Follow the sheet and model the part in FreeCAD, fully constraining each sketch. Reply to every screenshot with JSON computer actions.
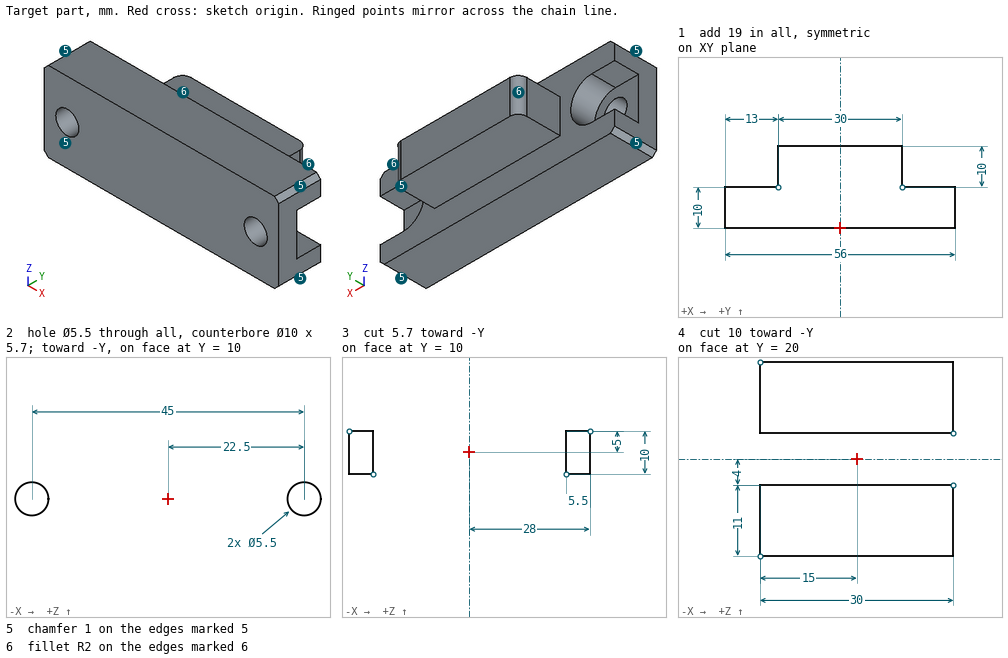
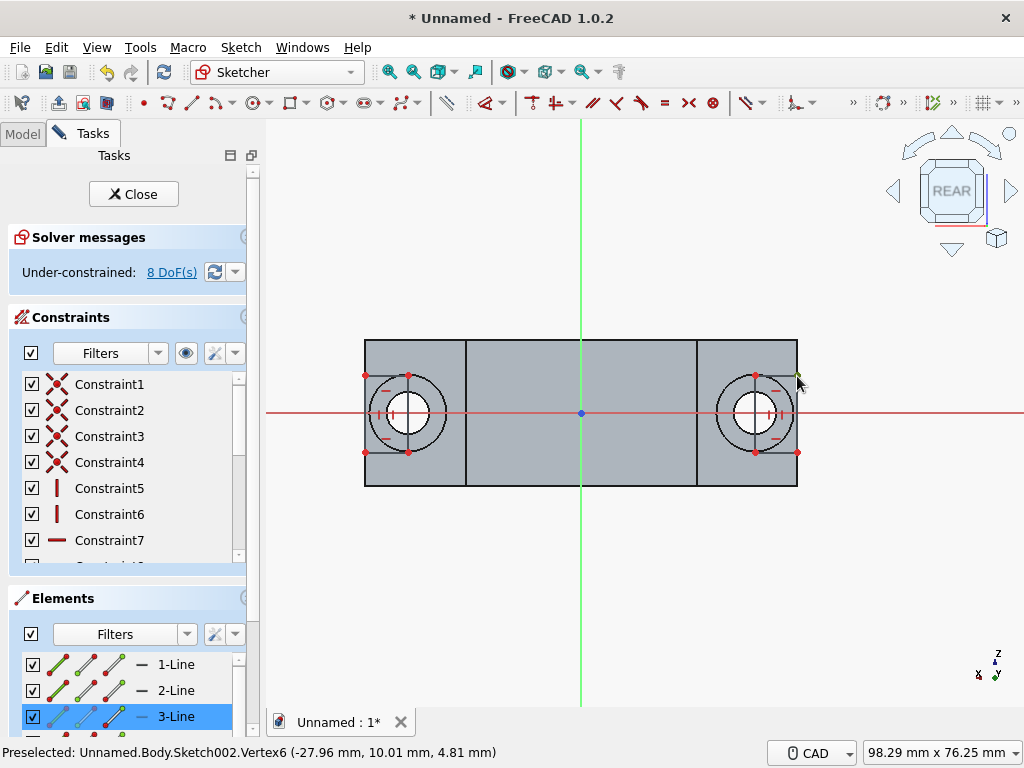
{"action": "left_click", "coordinate": [365, 376]}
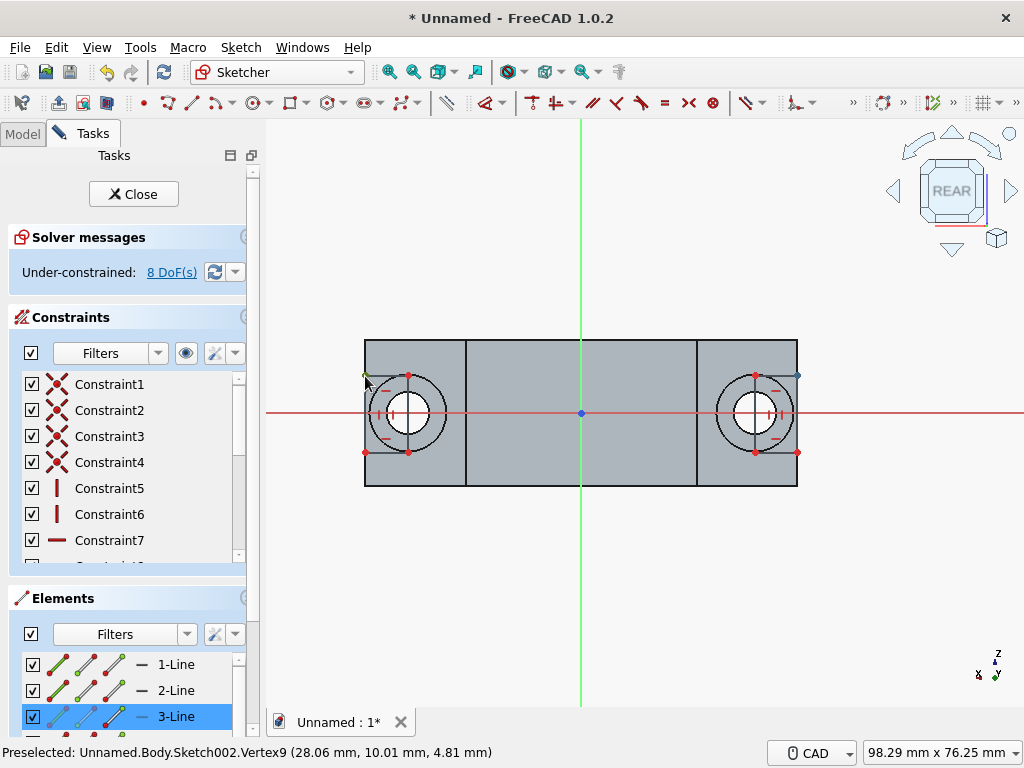
{"action": "left_click", "coordinate": [581, 641]}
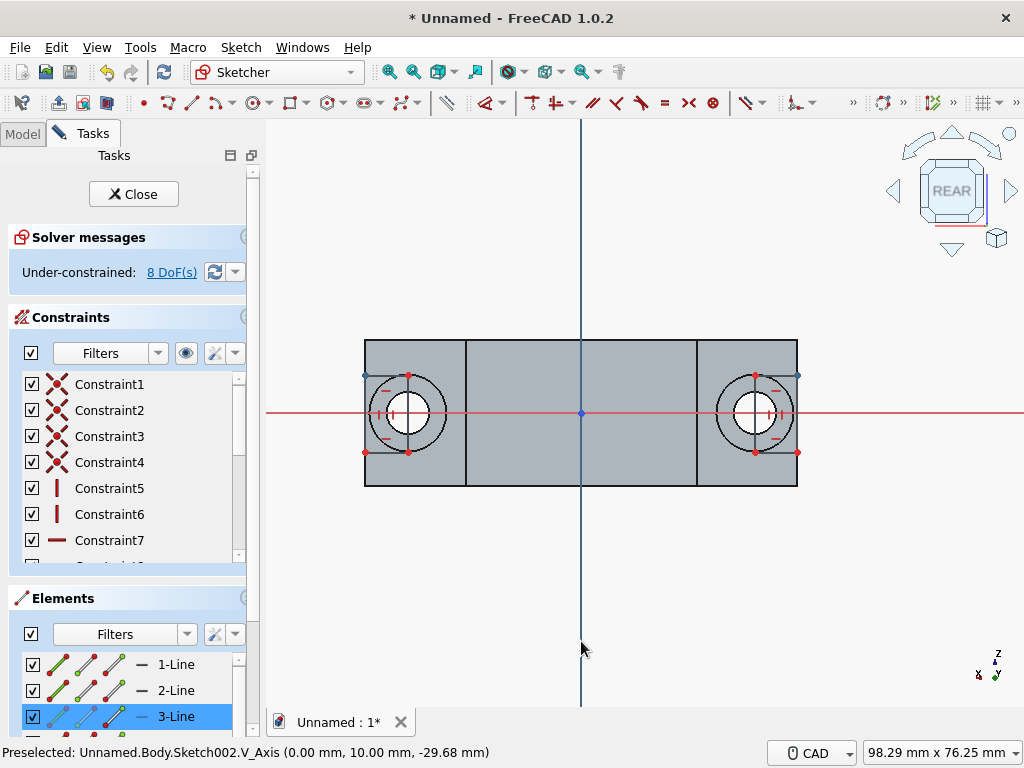
{"action": "left_click", "coordinate": [690, 104]}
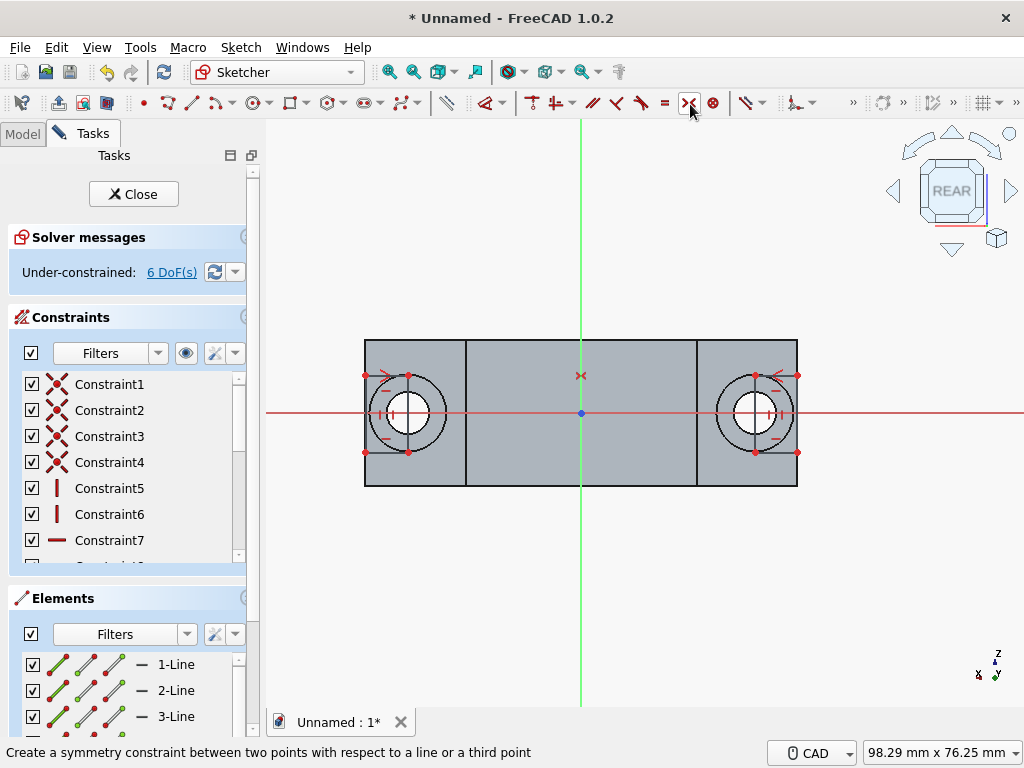
{"action": "left_click", "coordinate": [755, 453]}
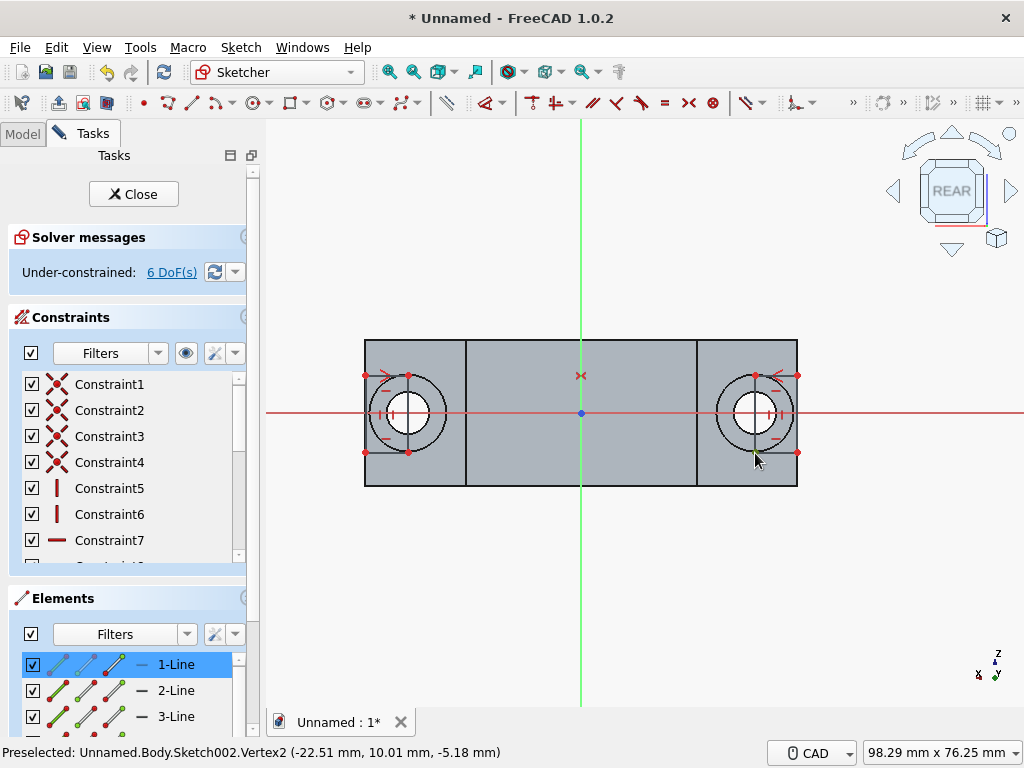
{"action": "left_click", "coordinate": [408, 453]}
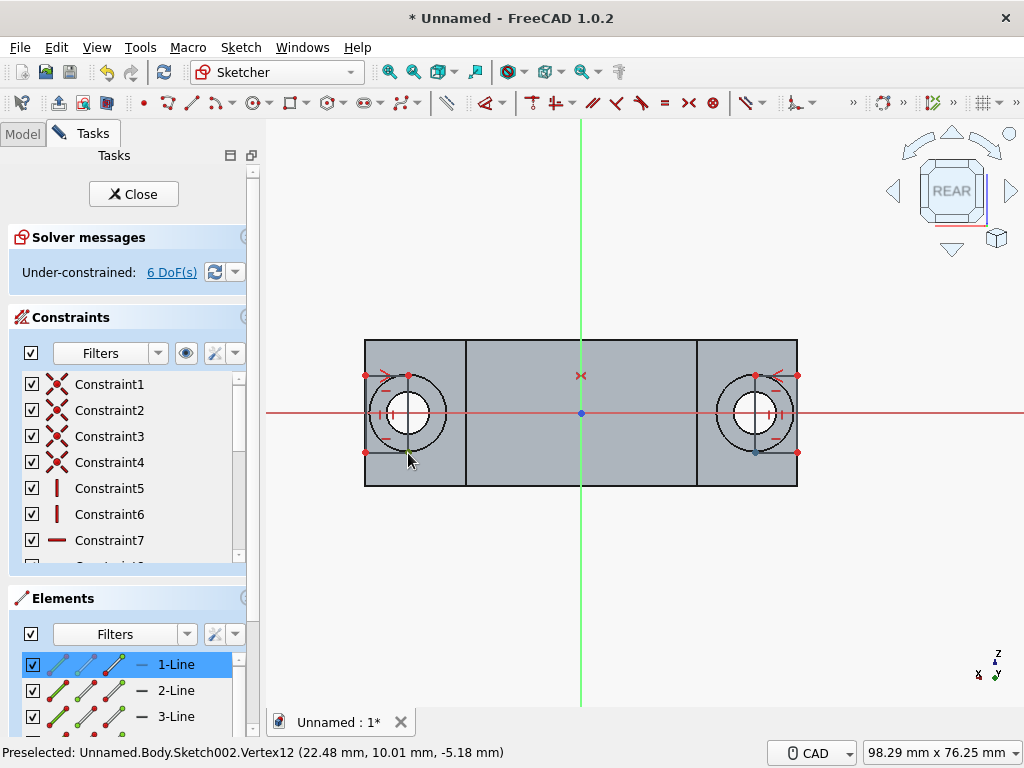
{"action": "left_click", "coordinate": [581, 641]}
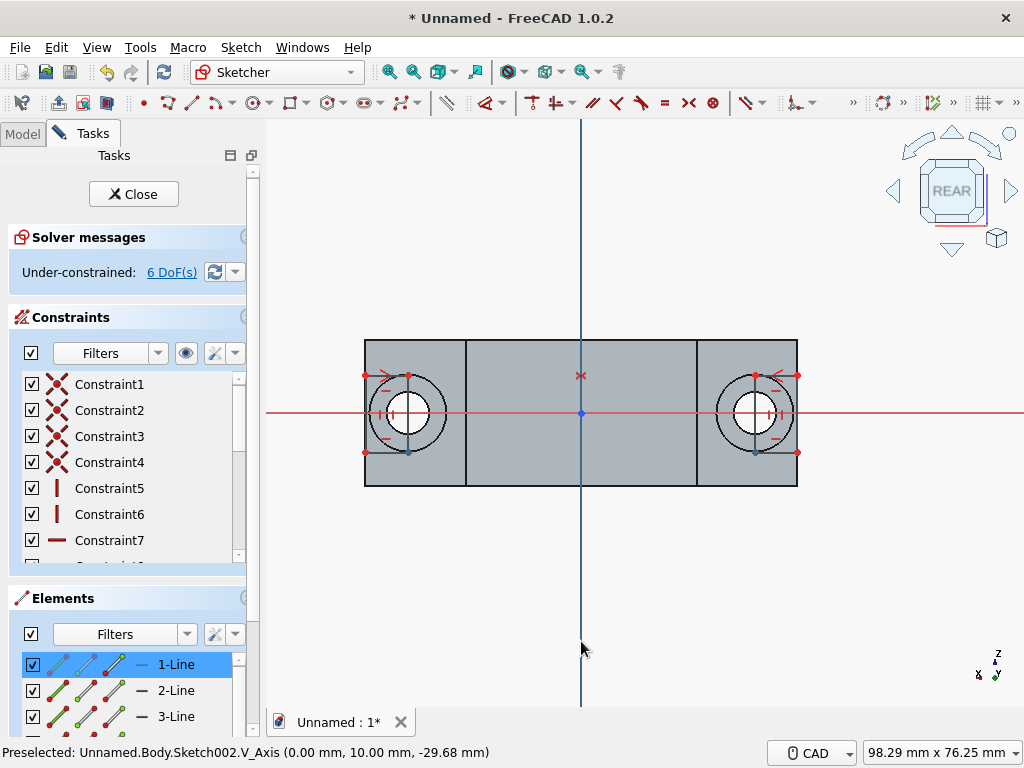
{"action": "left_click", "coordinate": [690, 104]}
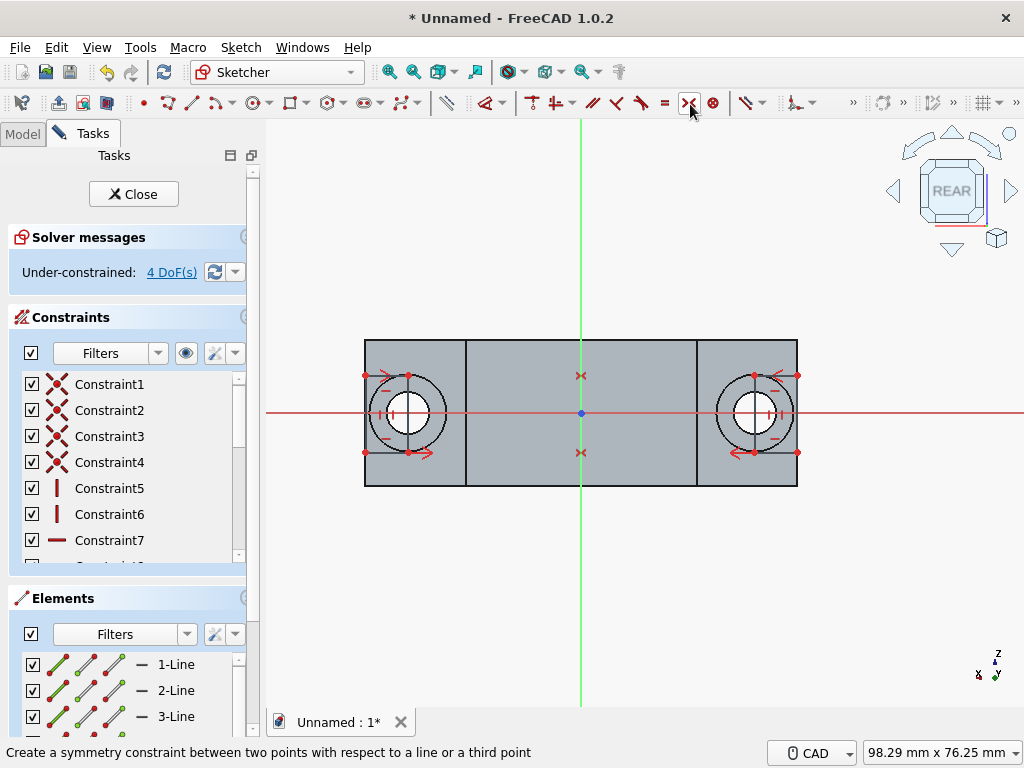
{"action": "left_click", "coordinate": [486, 104]}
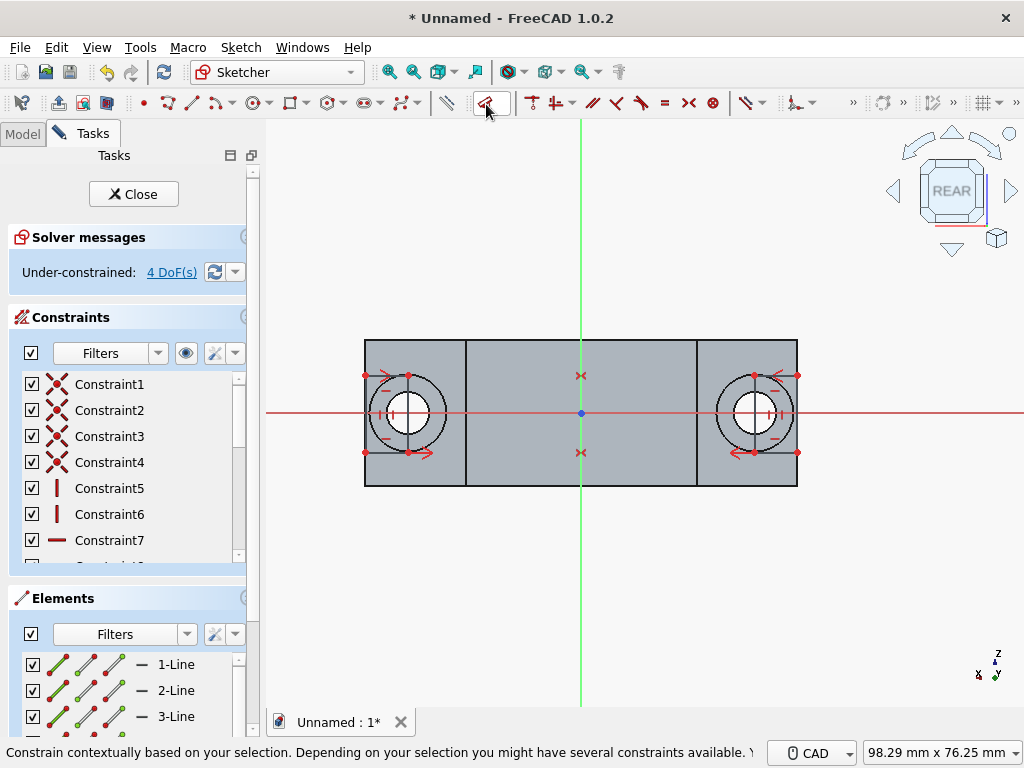
{"action": "left_click", "coordinate": [755, 399]}
{"action": "left_click", "coordinate": [721, 397]}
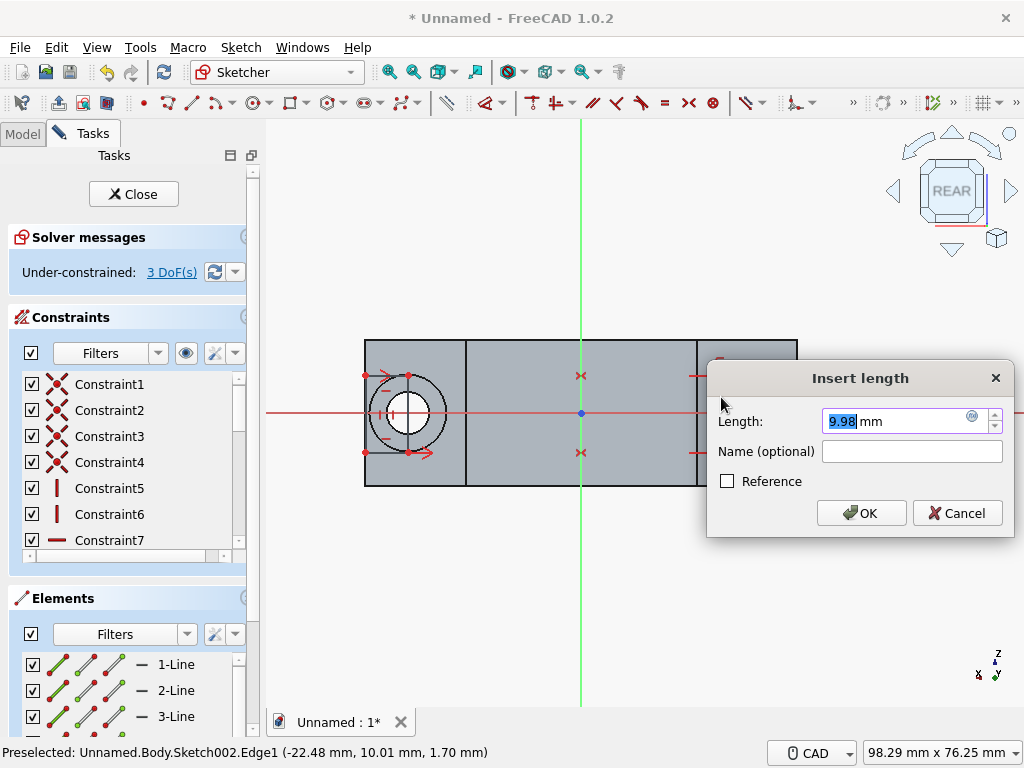
{"action": "type", "text": "10"}
{"action": "key", "text": "Return"}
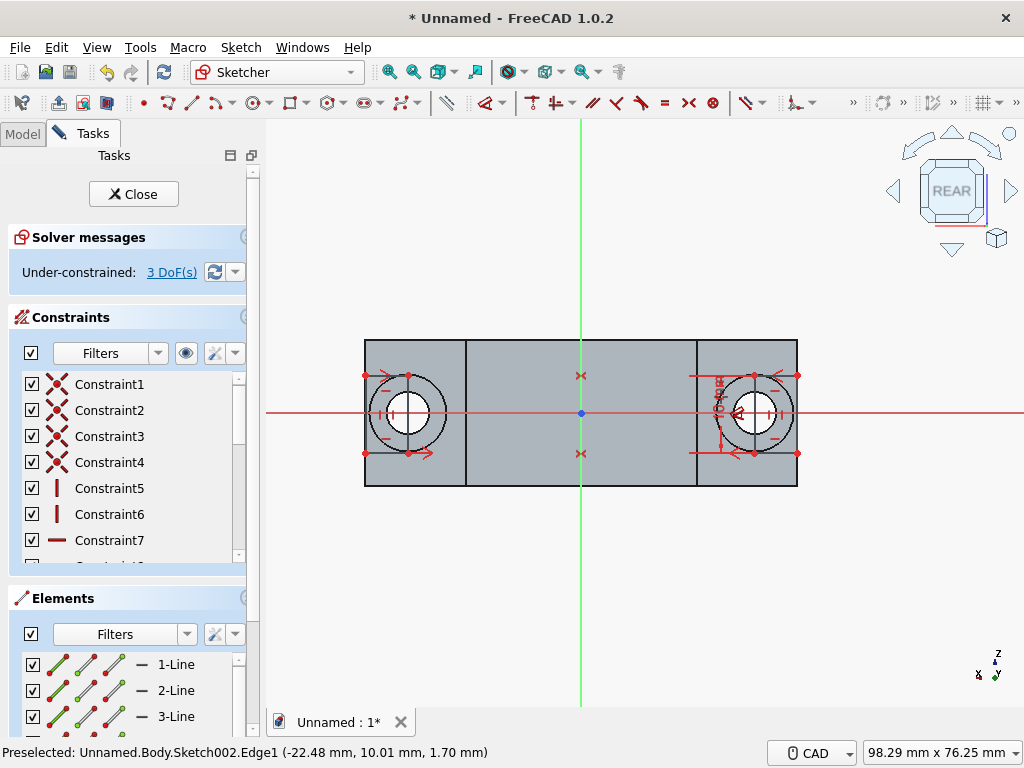
{"action": "left_click", "coordinate": [755, 376]}
{"action": "left_click", "coordinate": [547, 395]}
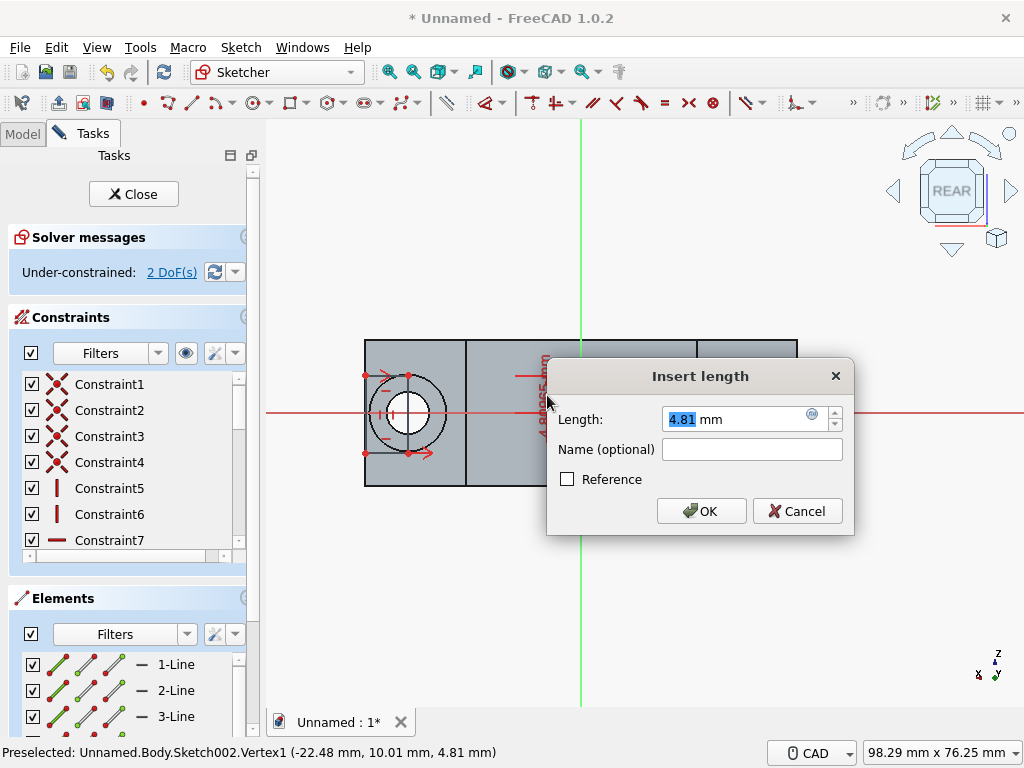
{"action": "type", "text": "5"}
{"action": "key", "text": "Return"}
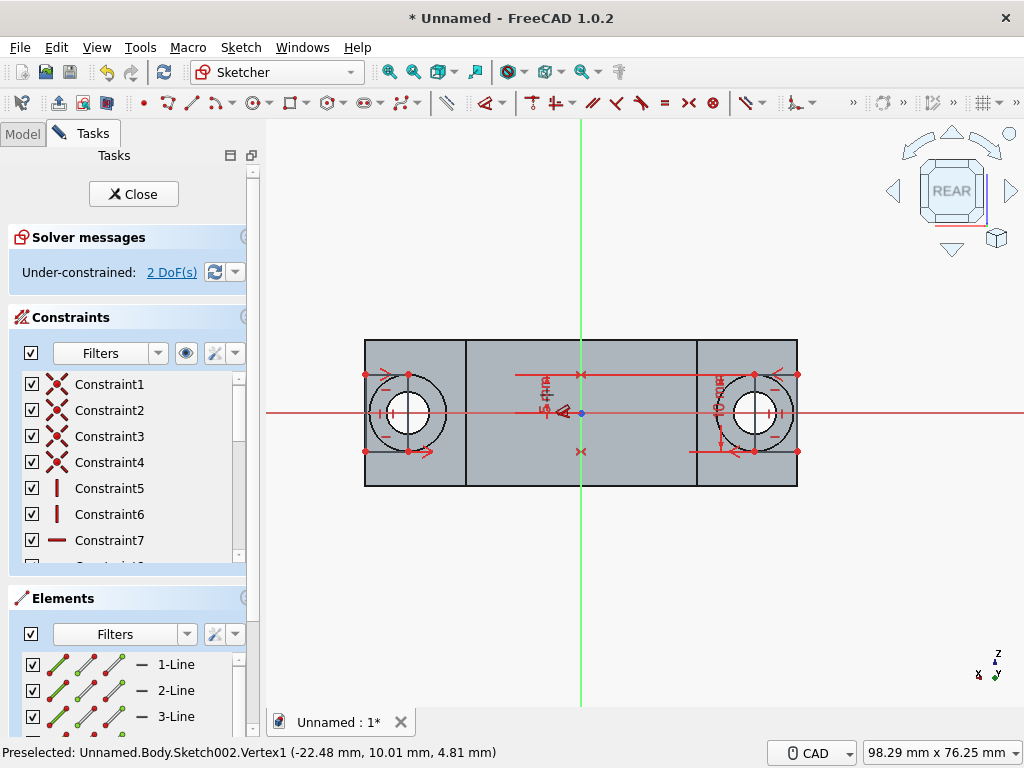
{"action": "left_click", "coordinate": [767, 452]}
{"action": "left_click", "coordinate": [776, 486]}